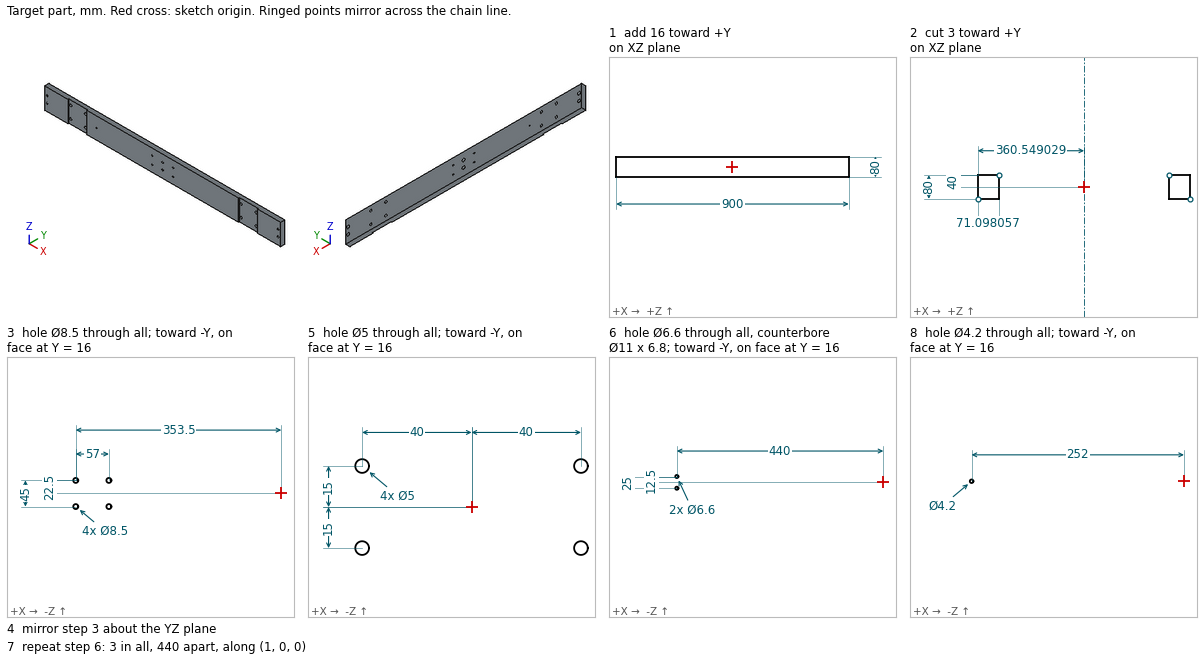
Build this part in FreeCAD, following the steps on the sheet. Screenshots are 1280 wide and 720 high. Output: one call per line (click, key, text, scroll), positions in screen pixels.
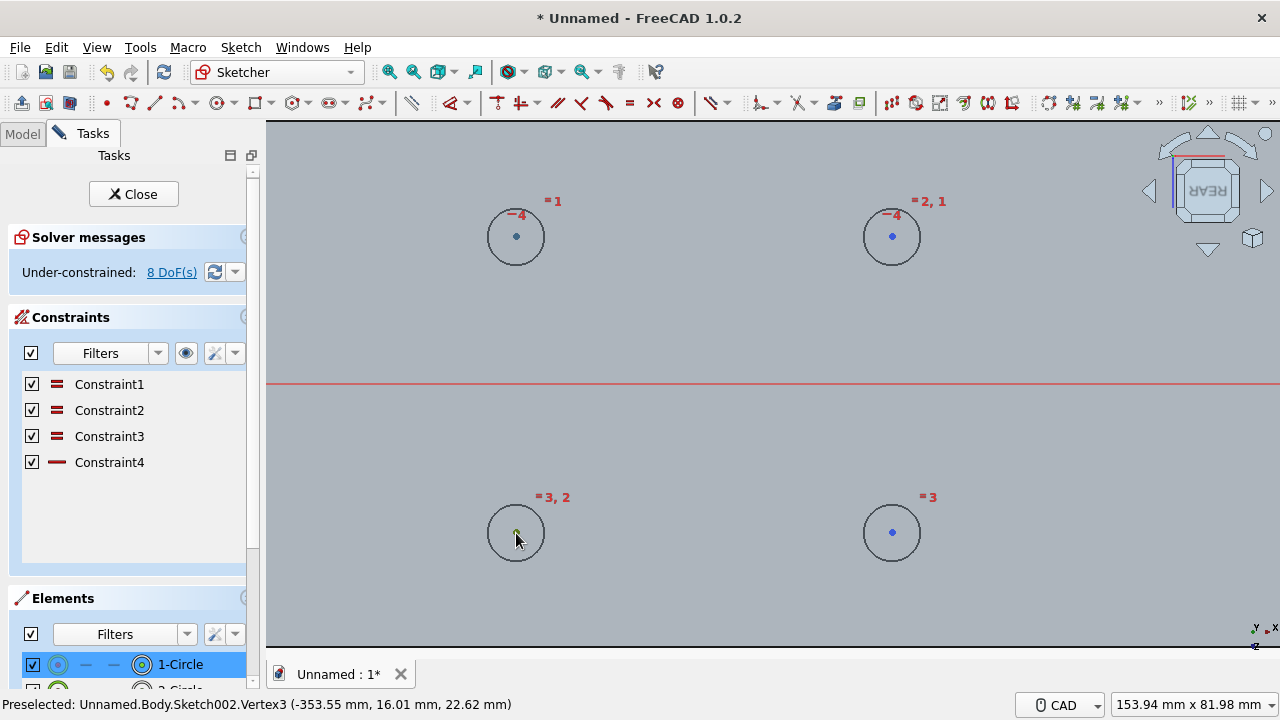
key(v)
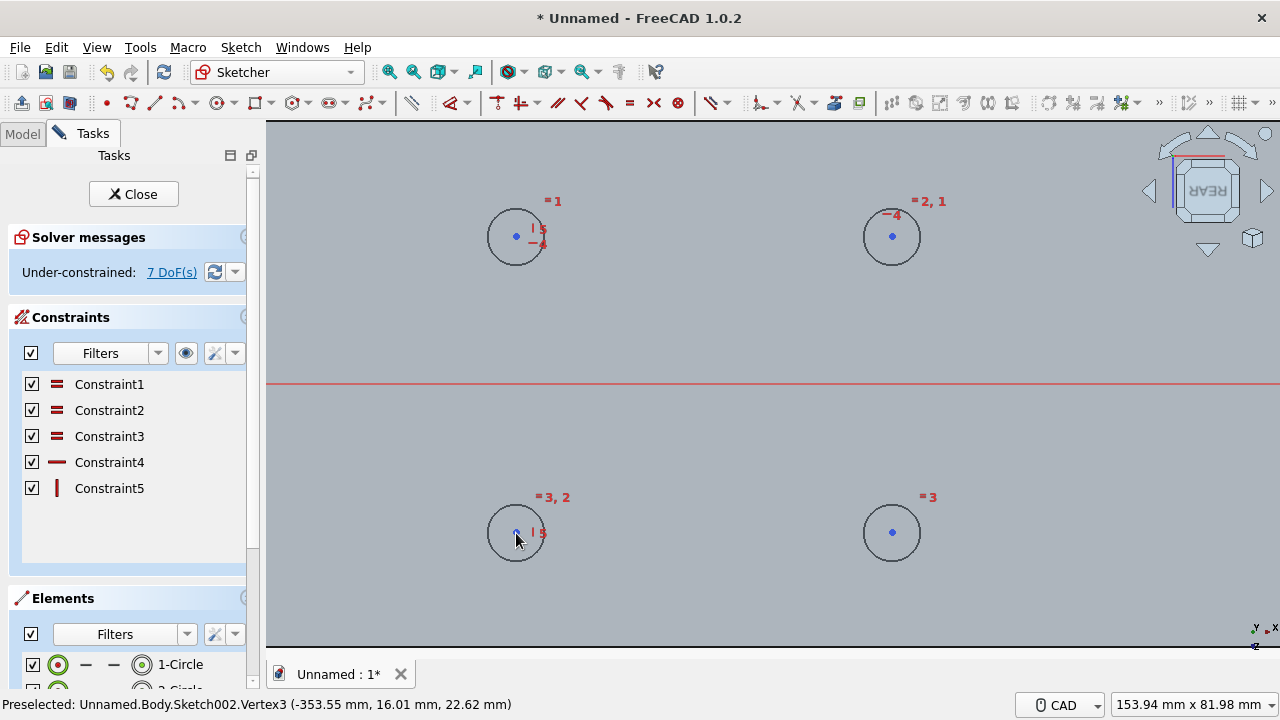
click(892, 237)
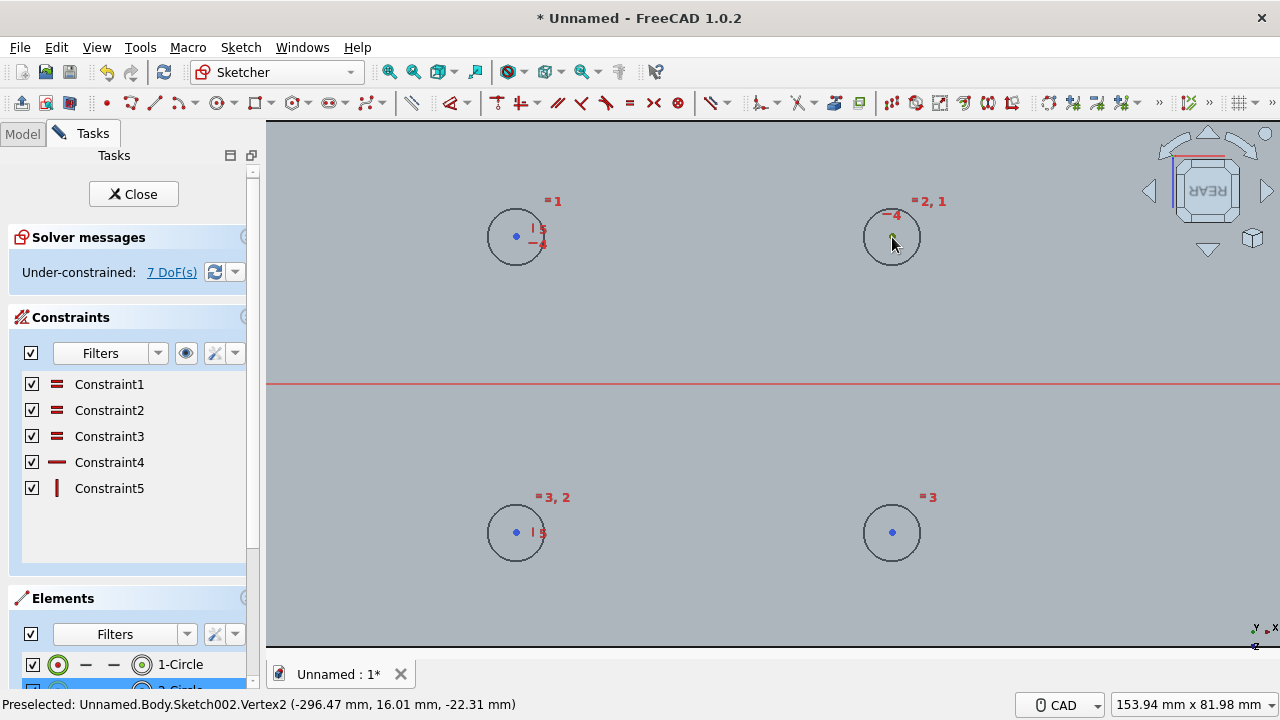
click(892, 533)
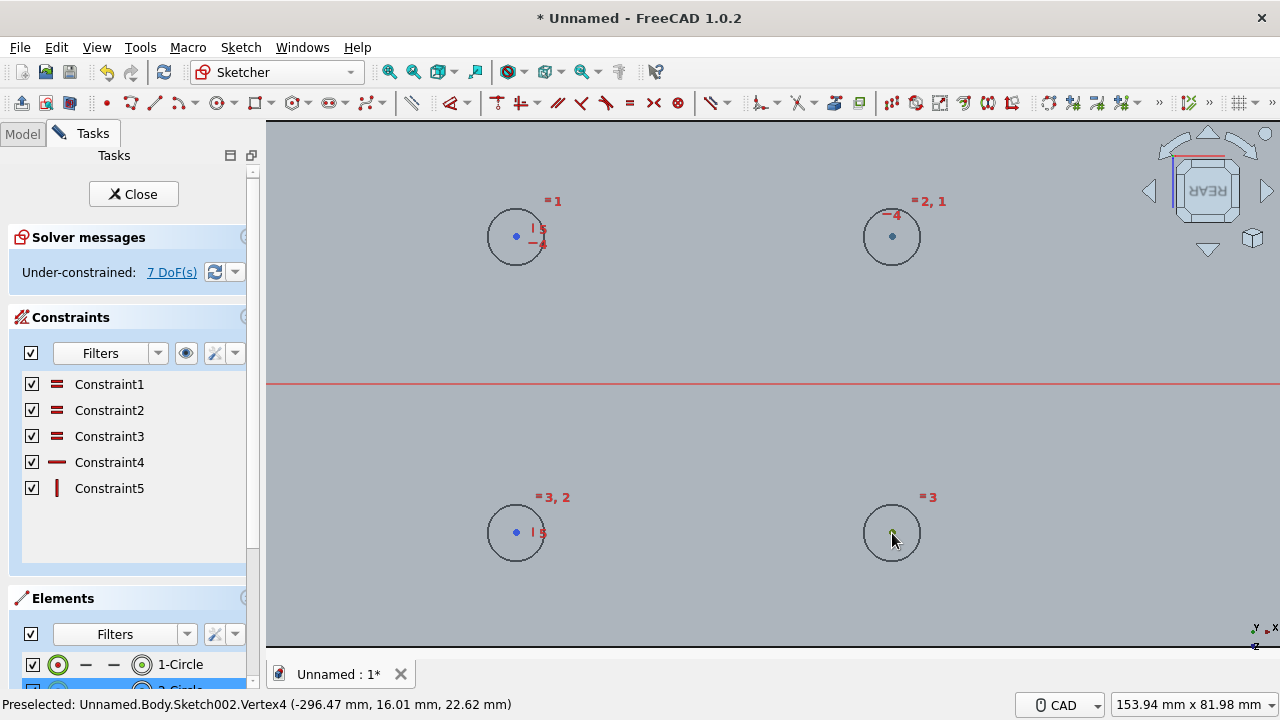
click(540, 104)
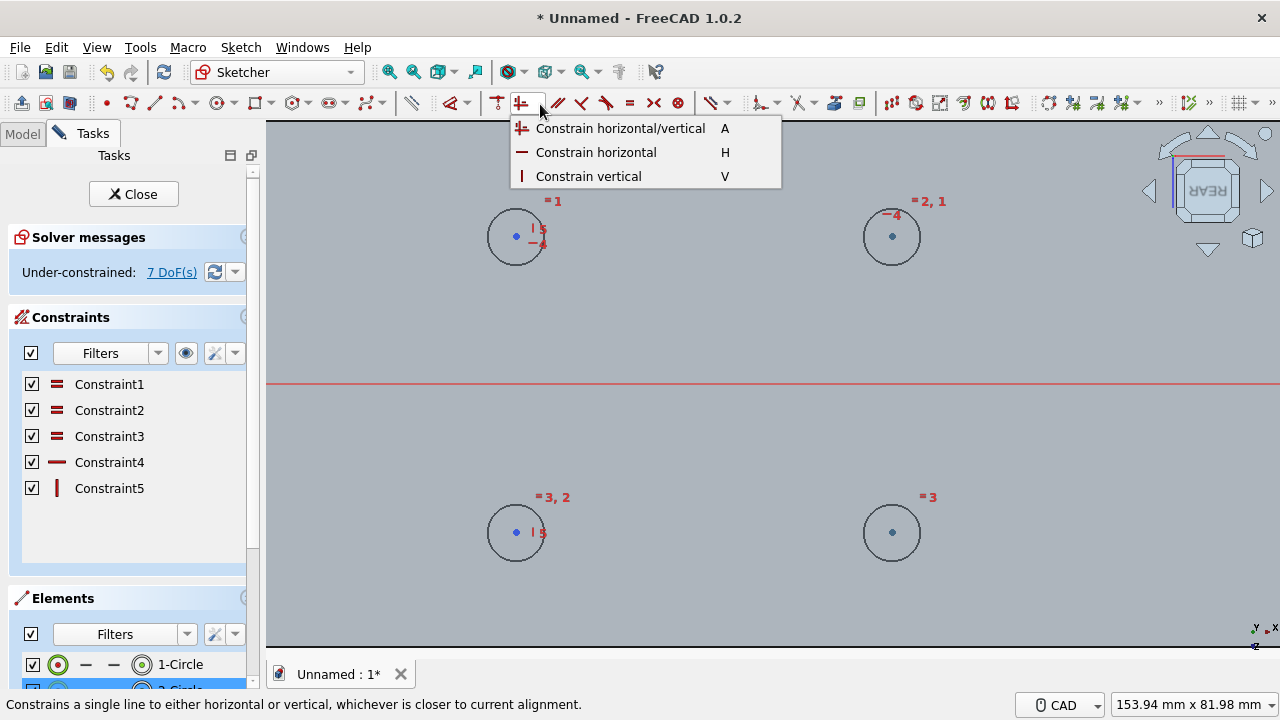
click(646, 176)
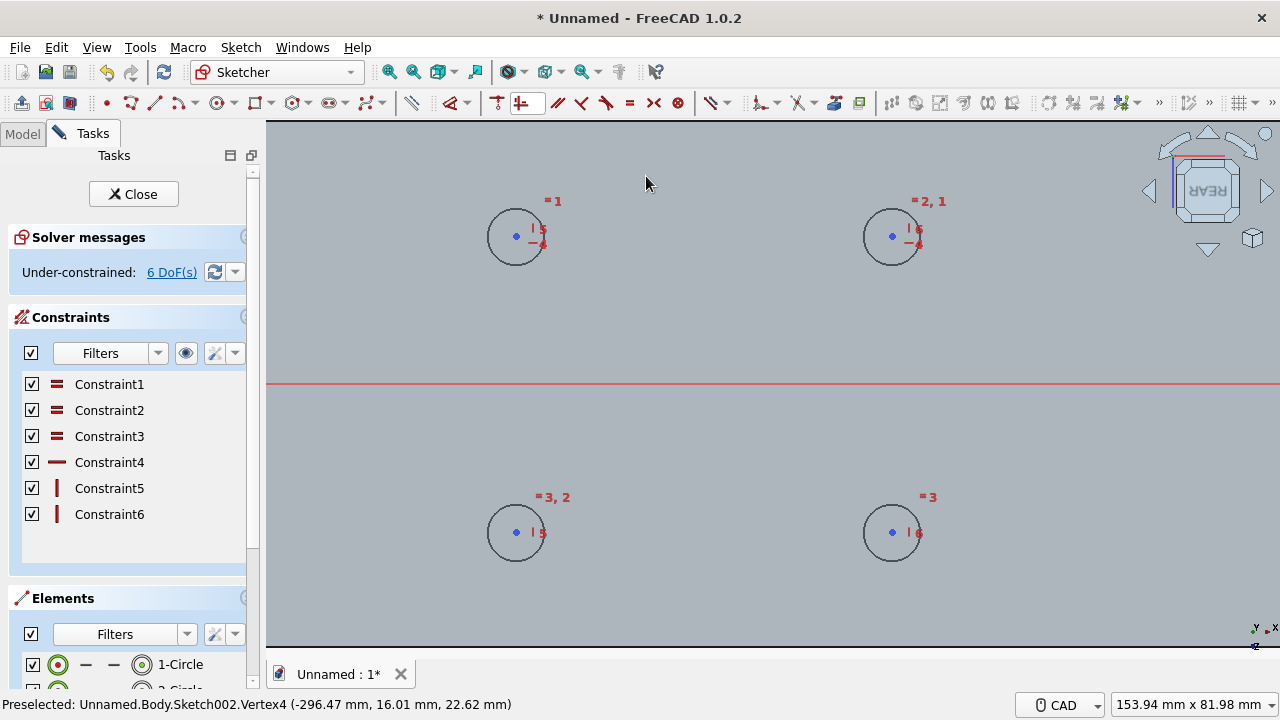
click(516, 533)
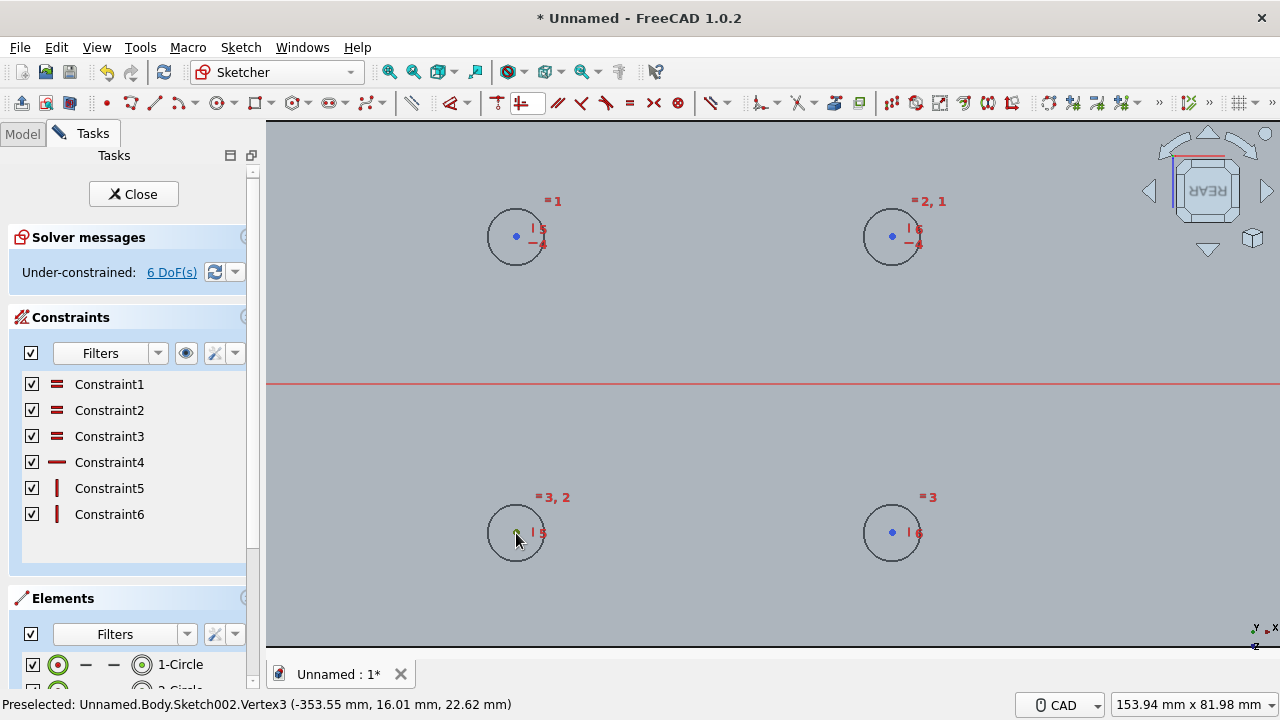
click(892, 533)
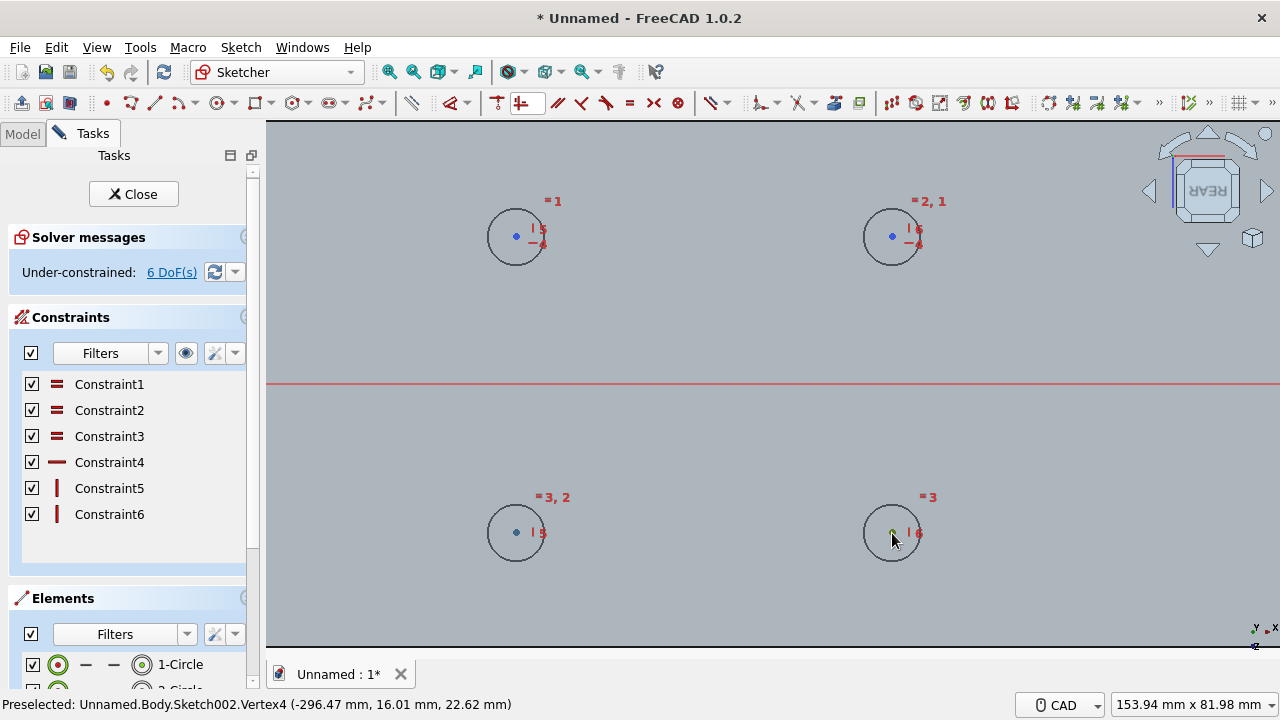
key(h)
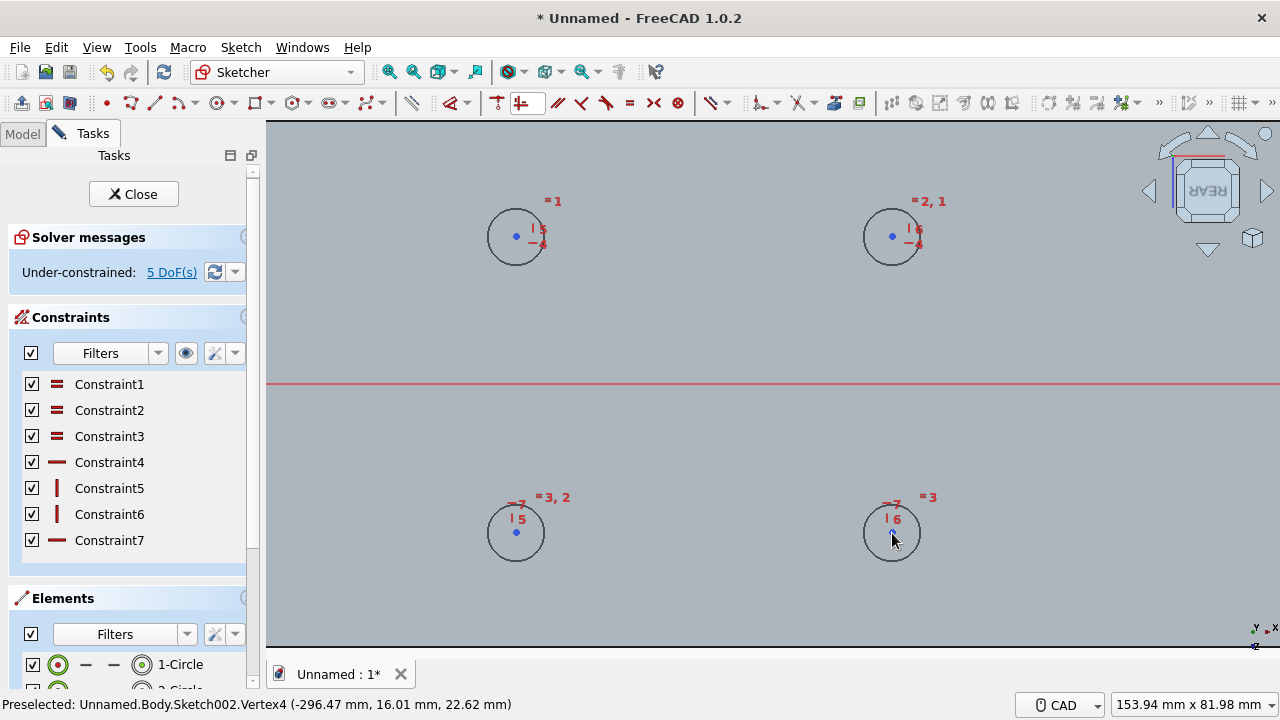
click(450, 104)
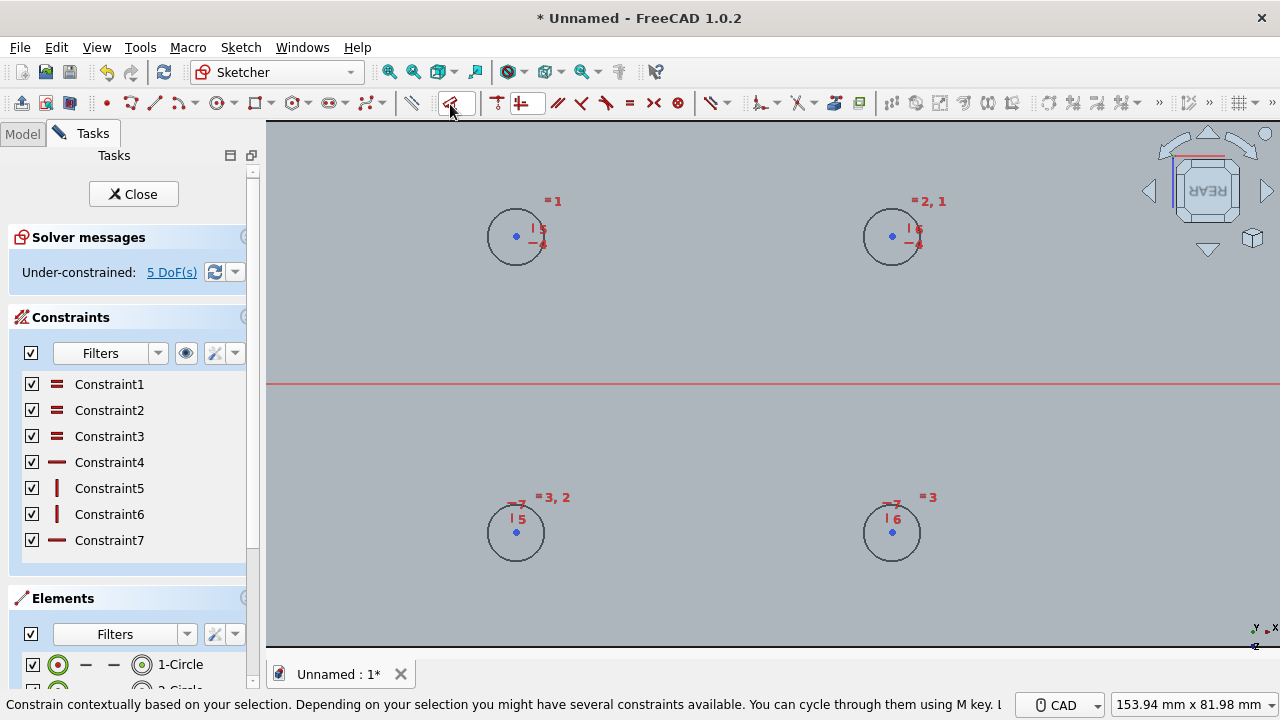
click(536, 217)
click(559, 194)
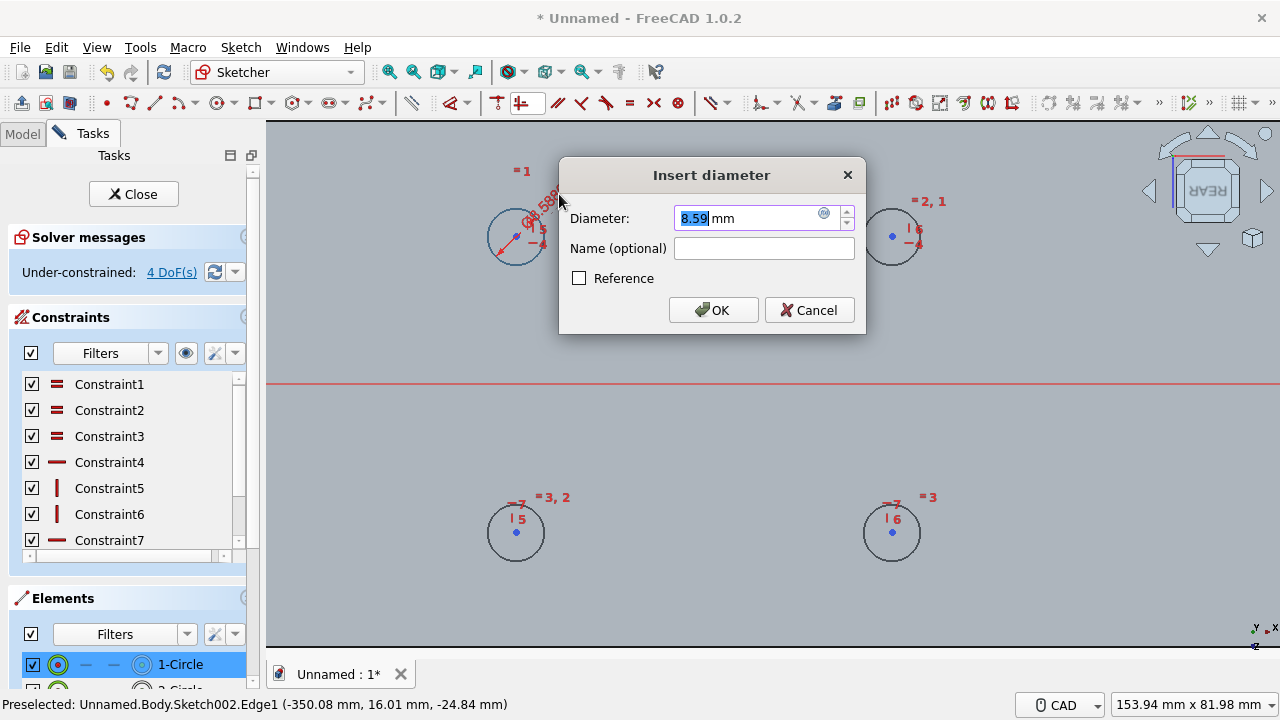
text(8.5)
key(Return)